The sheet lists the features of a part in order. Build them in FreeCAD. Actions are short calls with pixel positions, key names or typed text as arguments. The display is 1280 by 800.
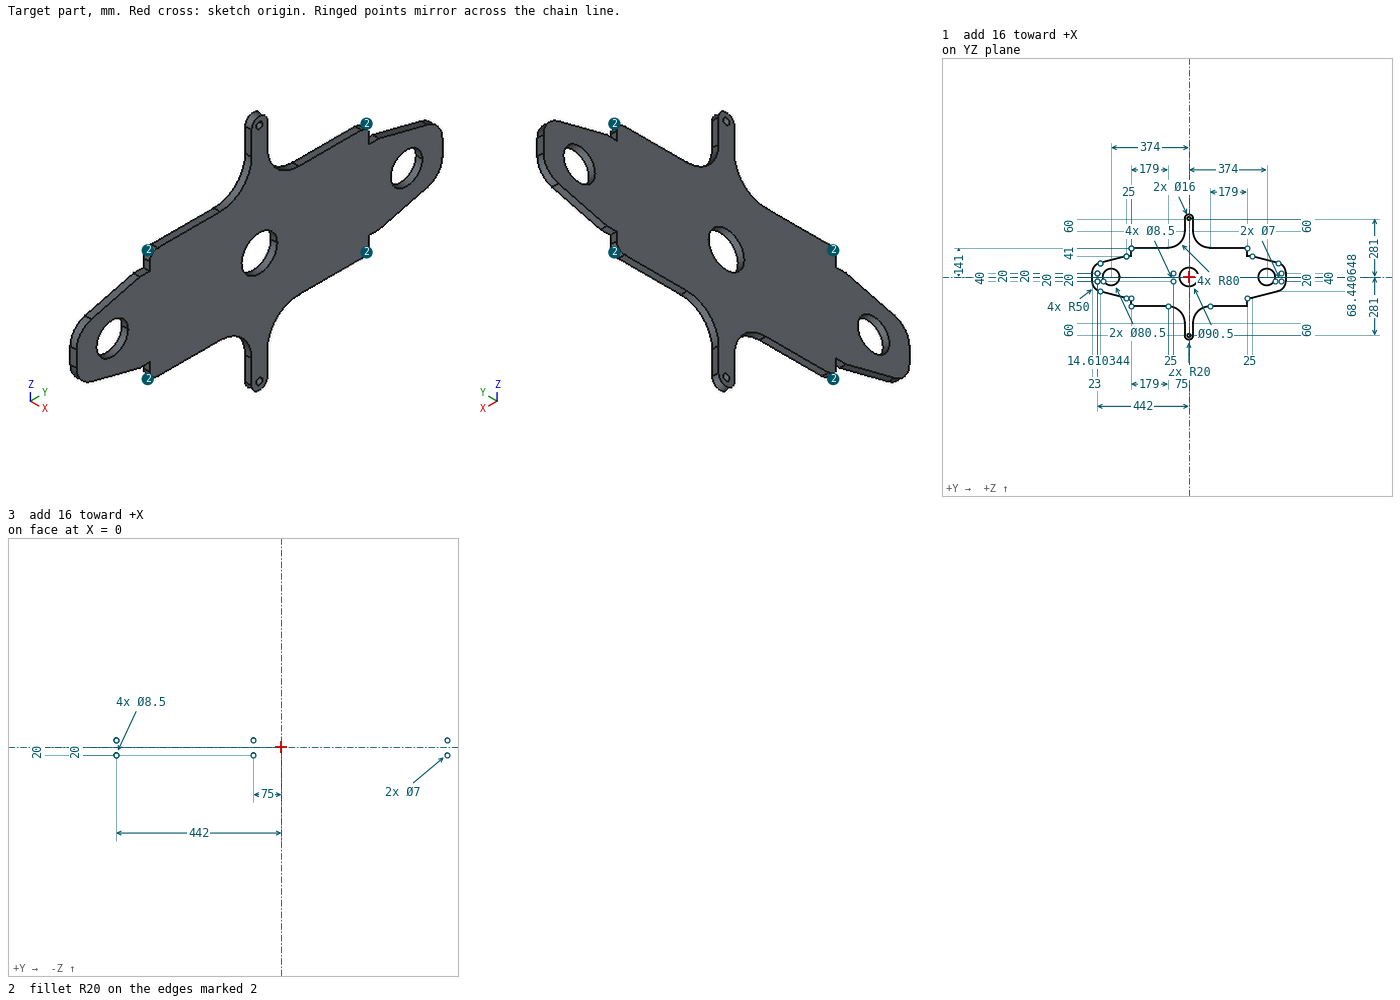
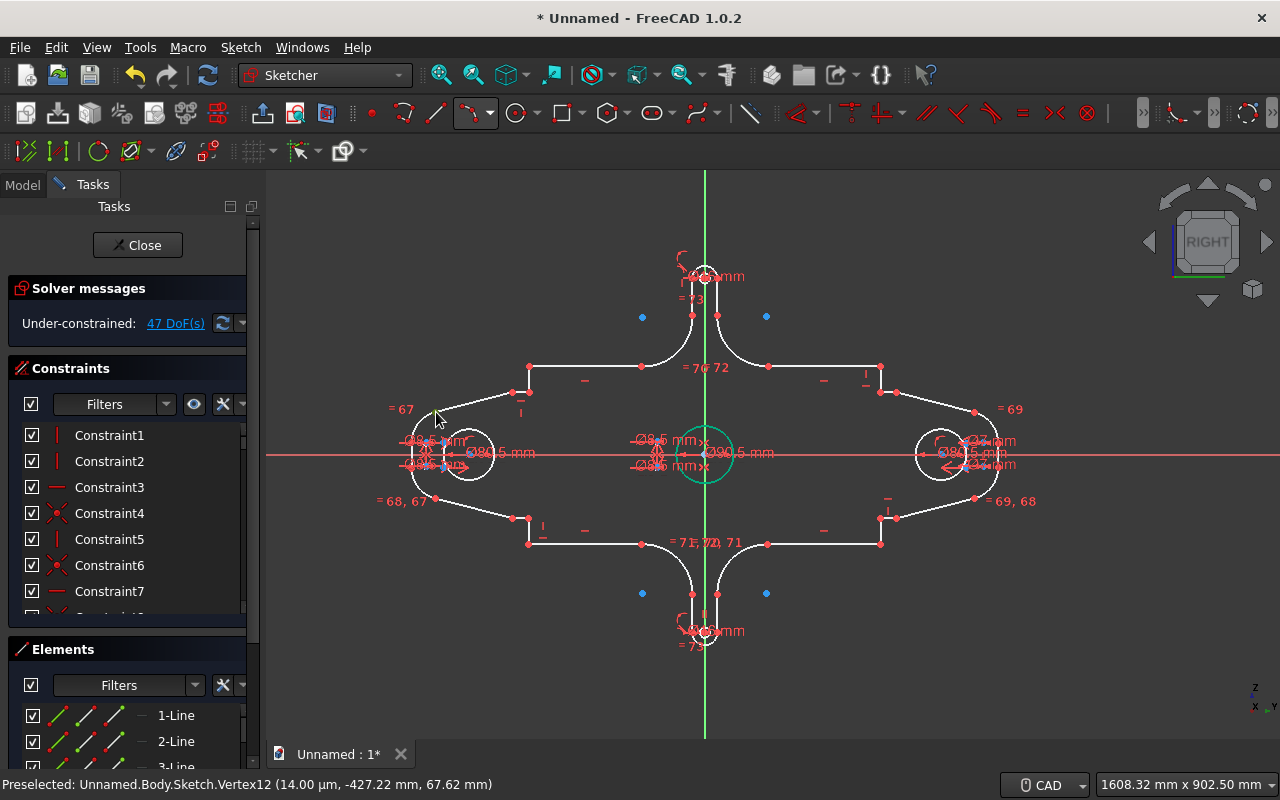
click(435, 498)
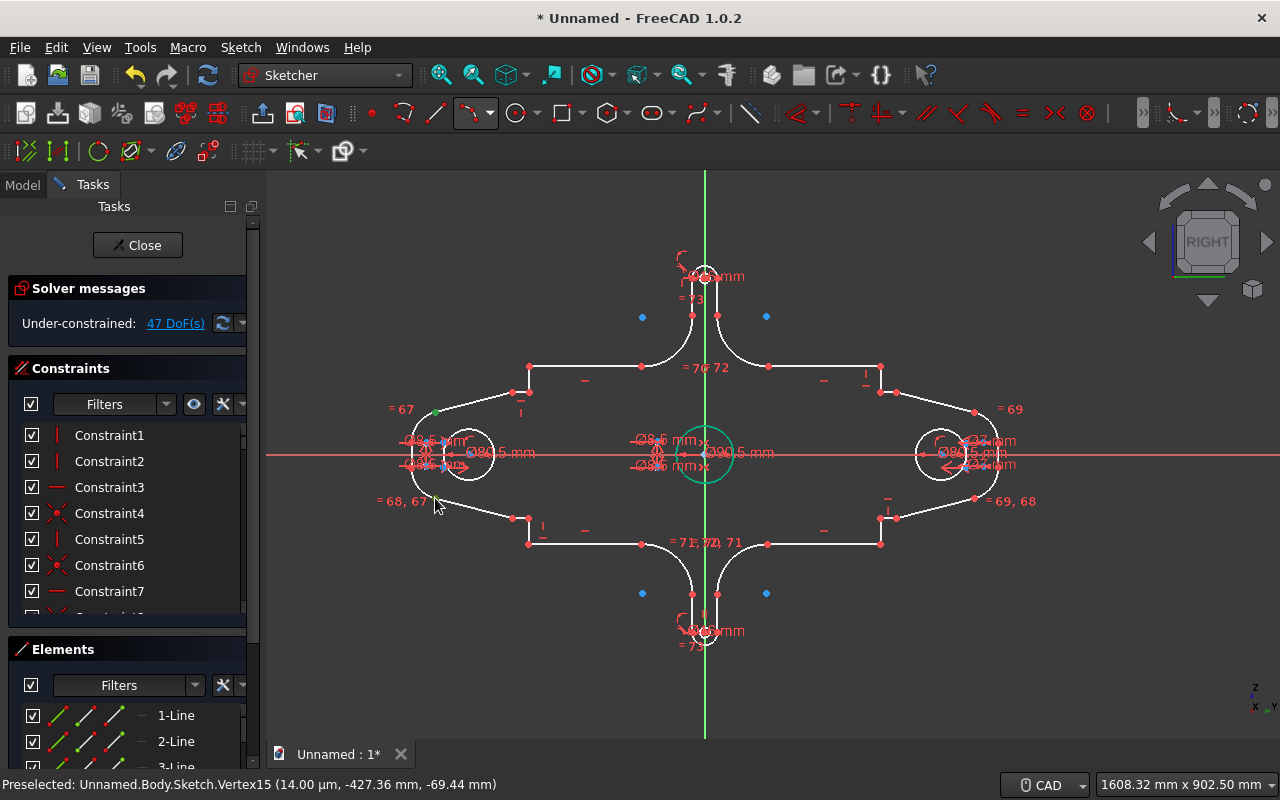
click(353, 455)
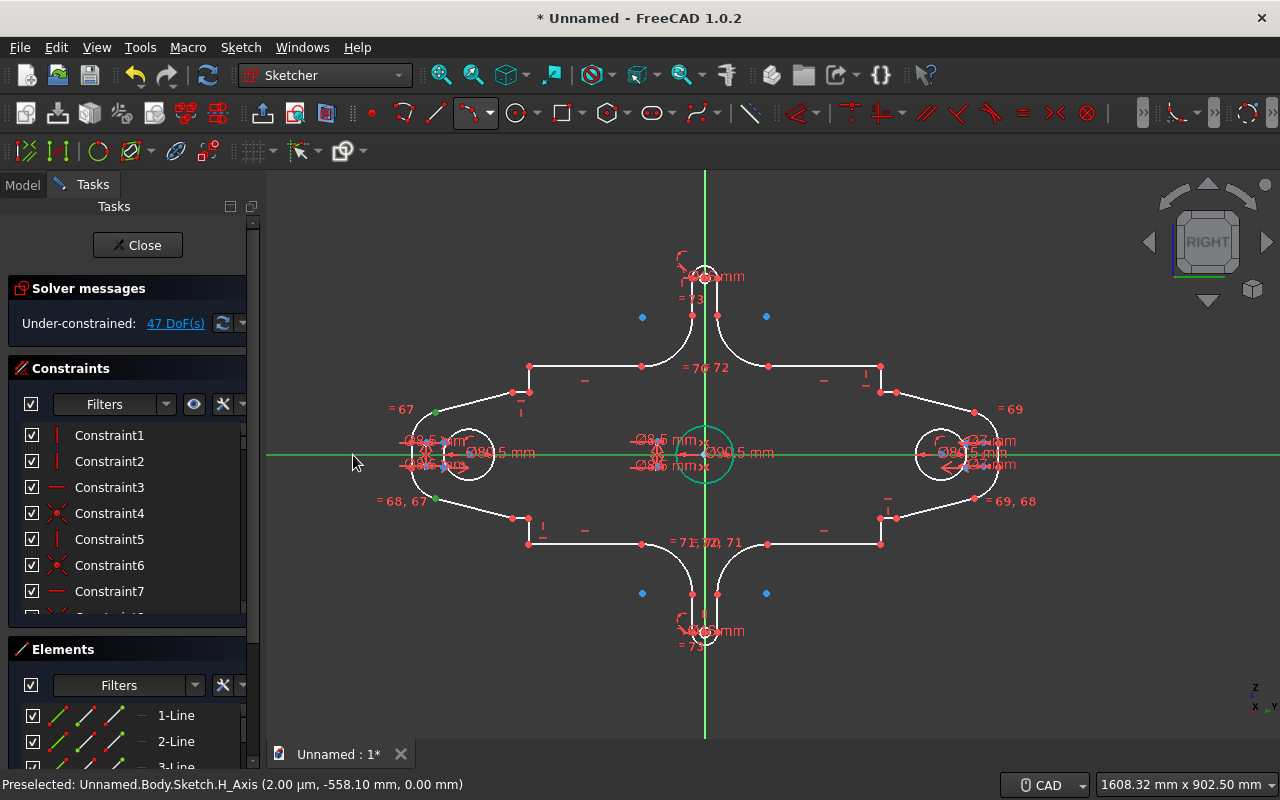
click(1056, 114)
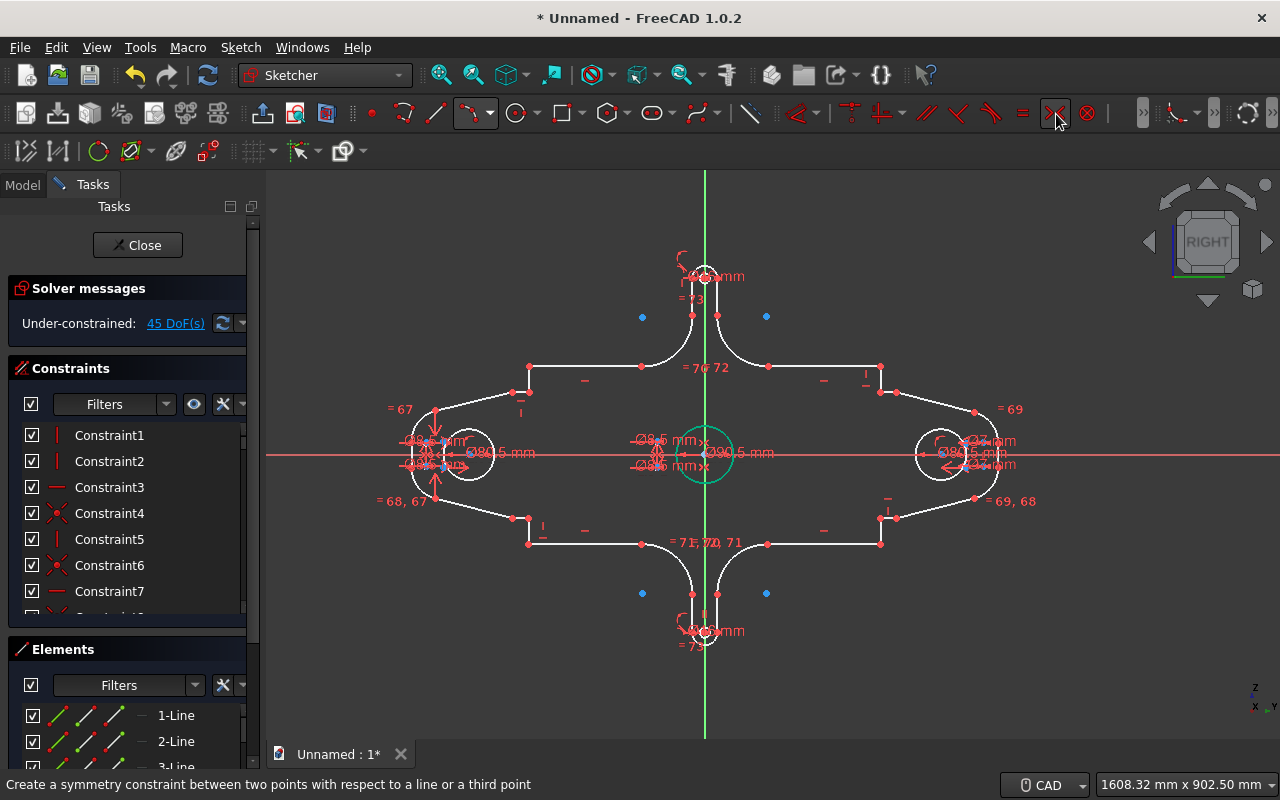
click(513, 392)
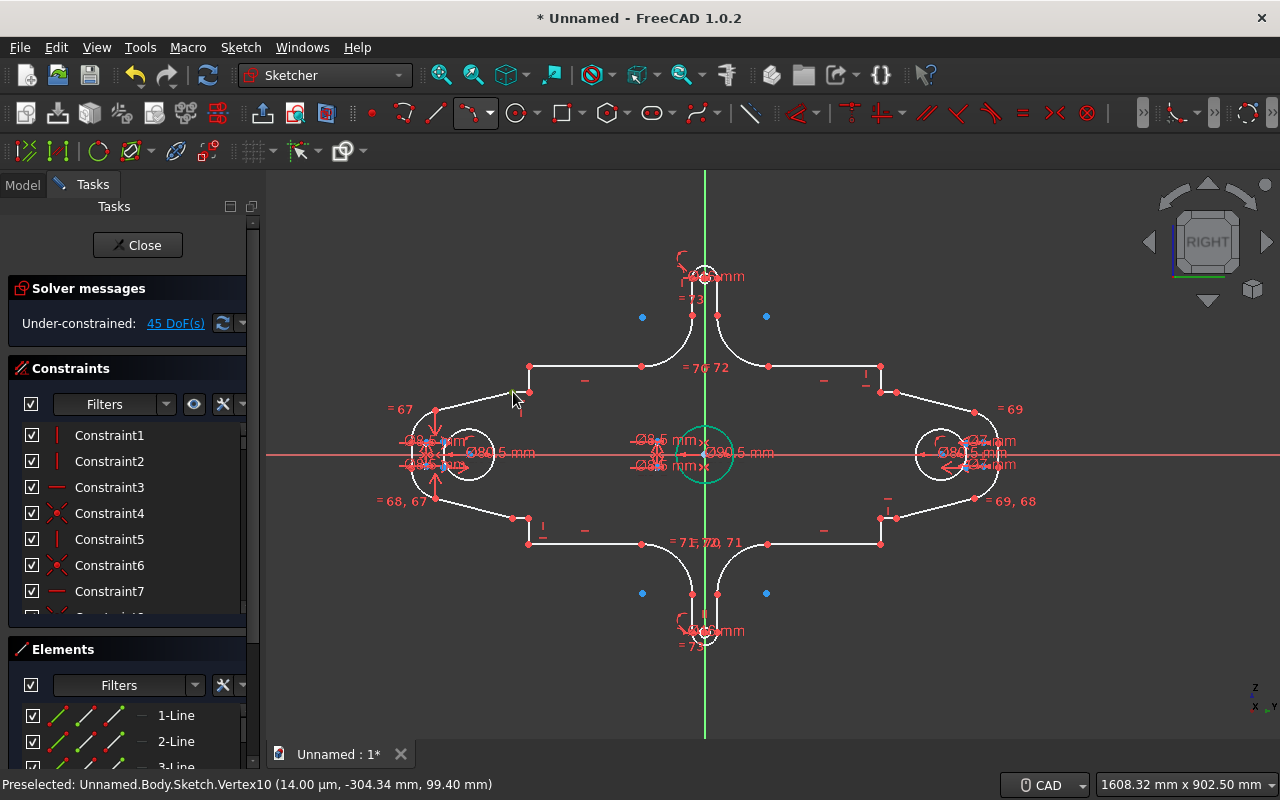
click(513, 518)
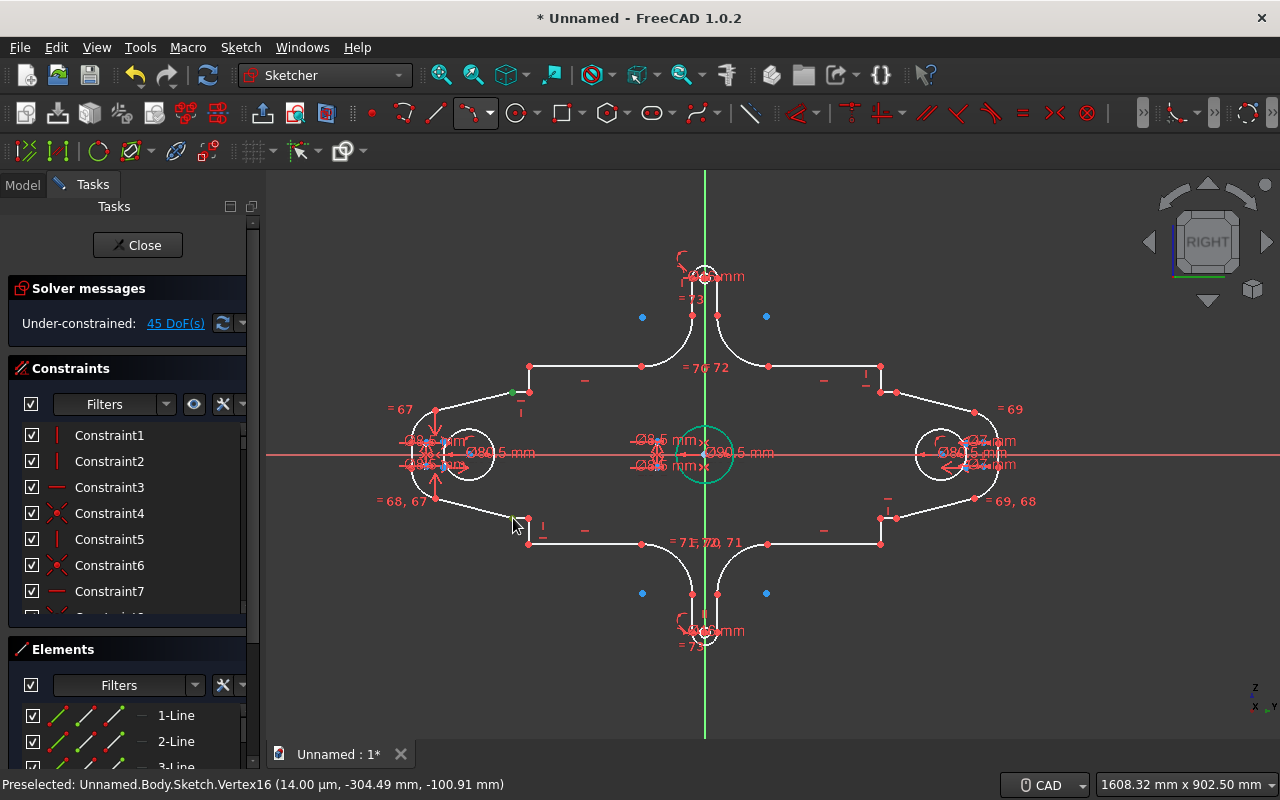
click(353, 455)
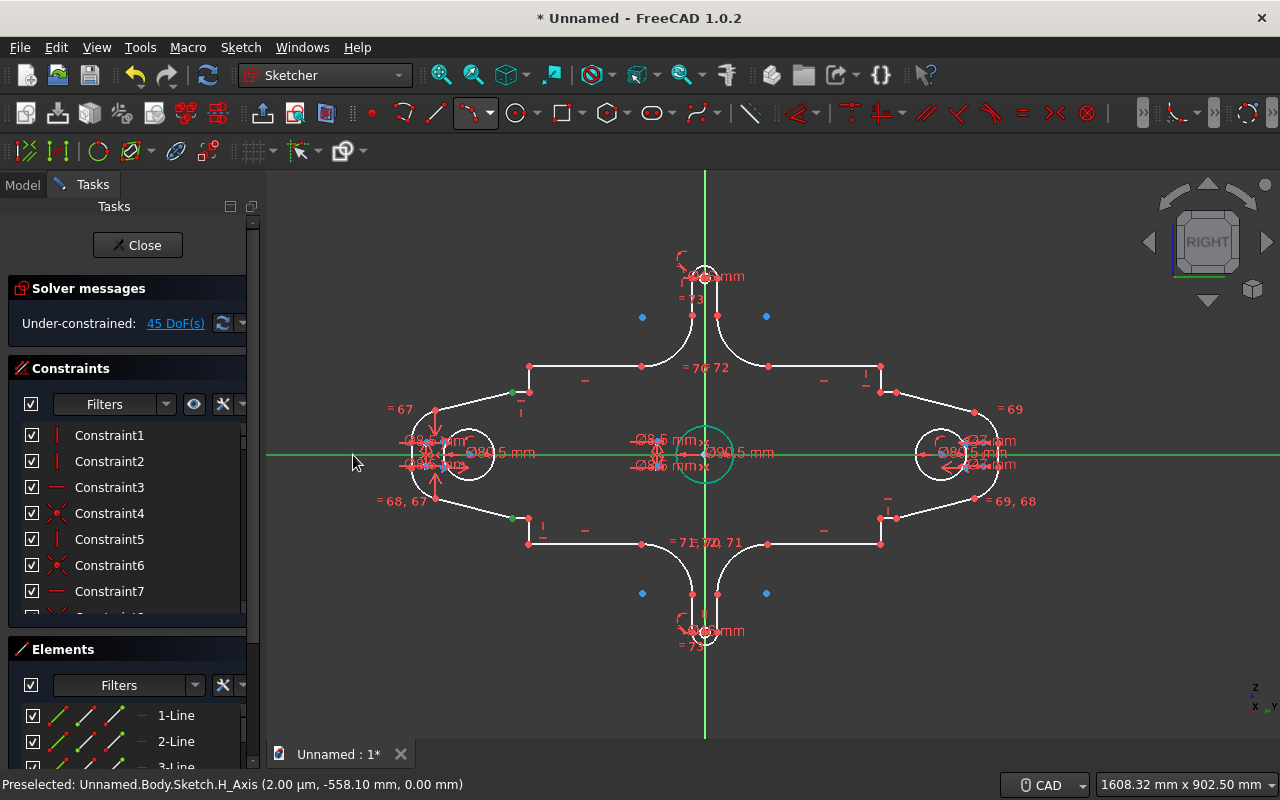
key(s)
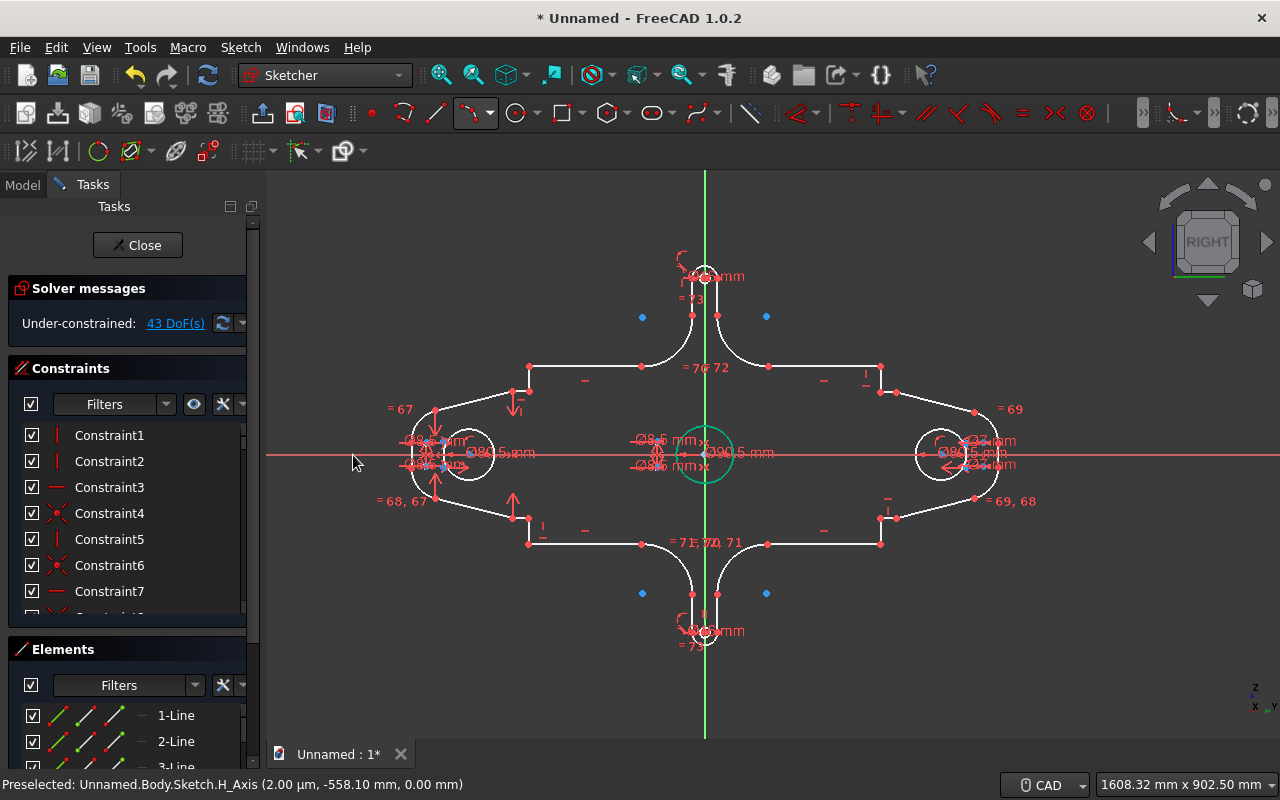
click(529, 366)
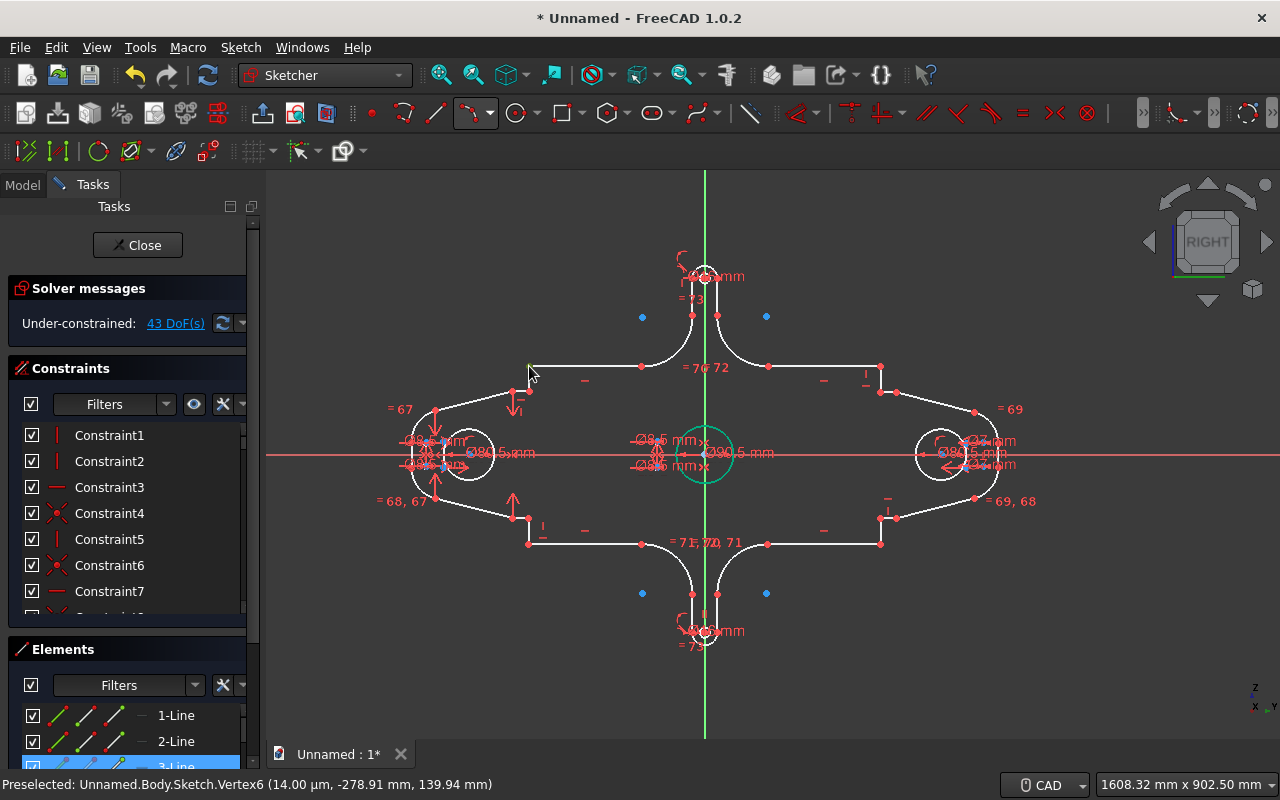
click(529, 544)